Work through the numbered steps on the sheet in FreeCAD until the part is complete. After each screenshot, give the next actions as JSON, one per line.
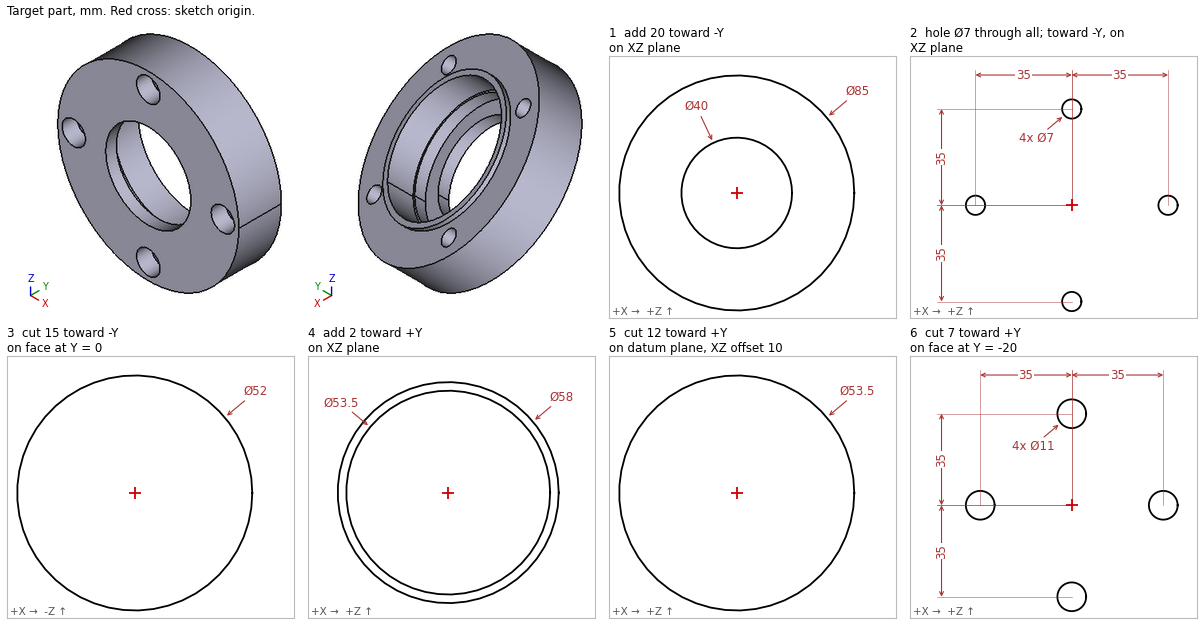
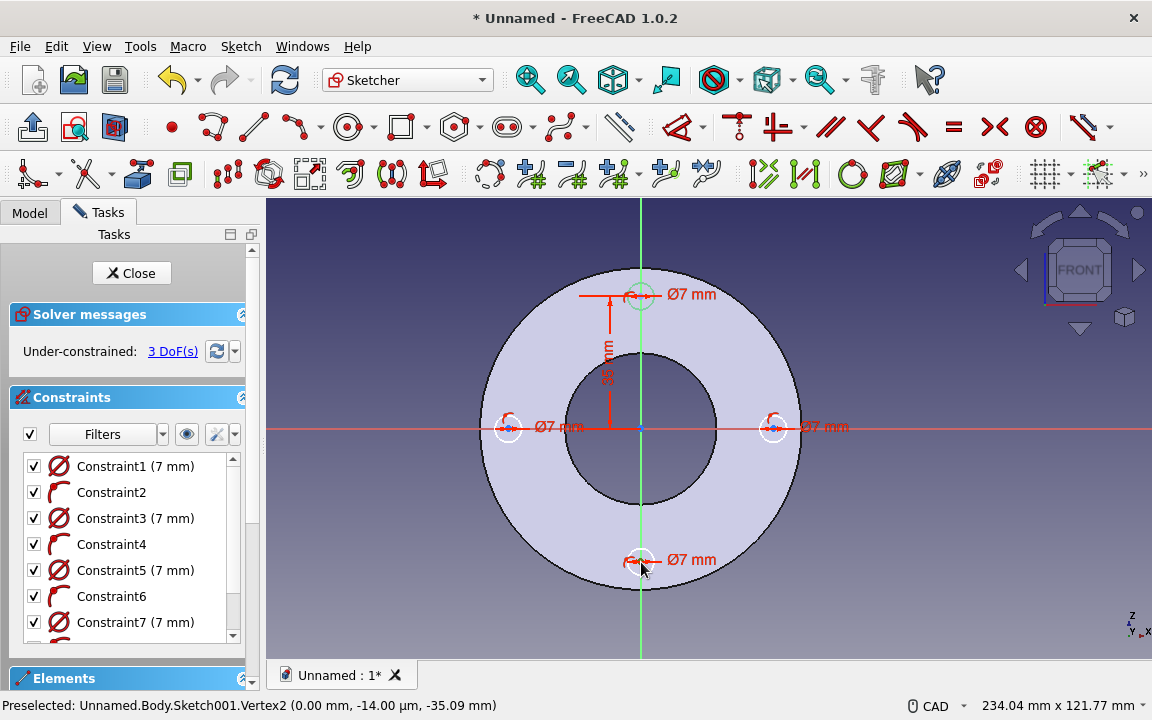
{"action": "key", "text": "i"}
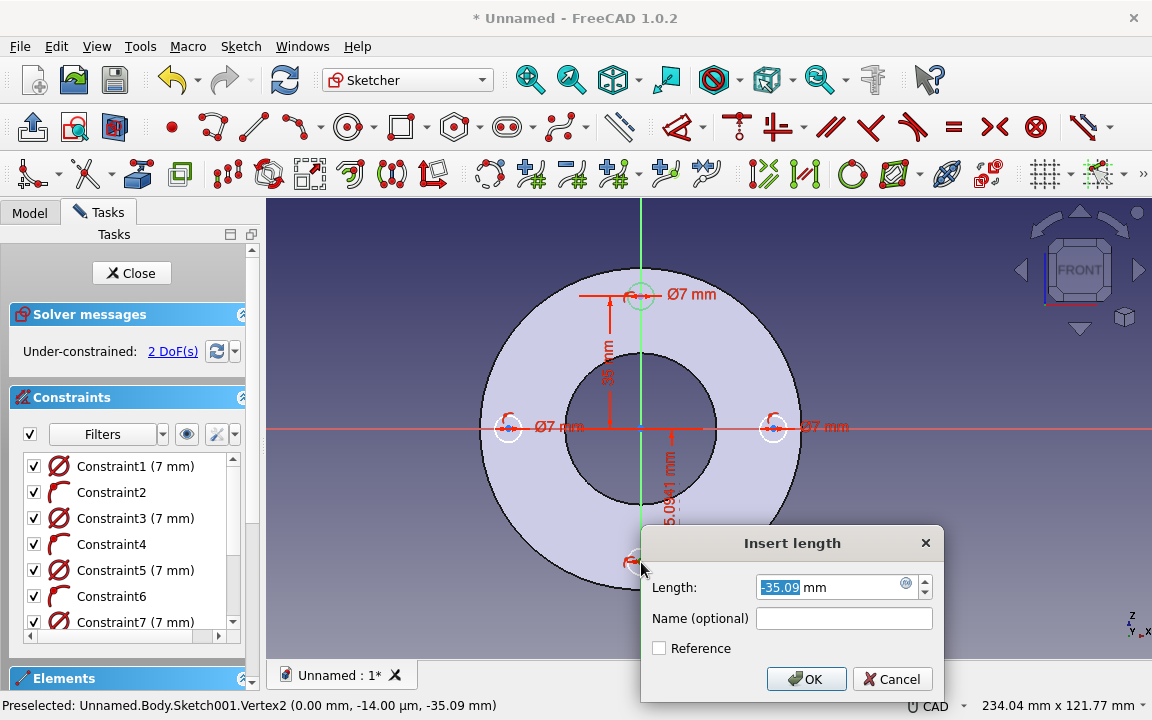
{"action": "type", "text": "-35"}
{"action": "key", "text": "Return"}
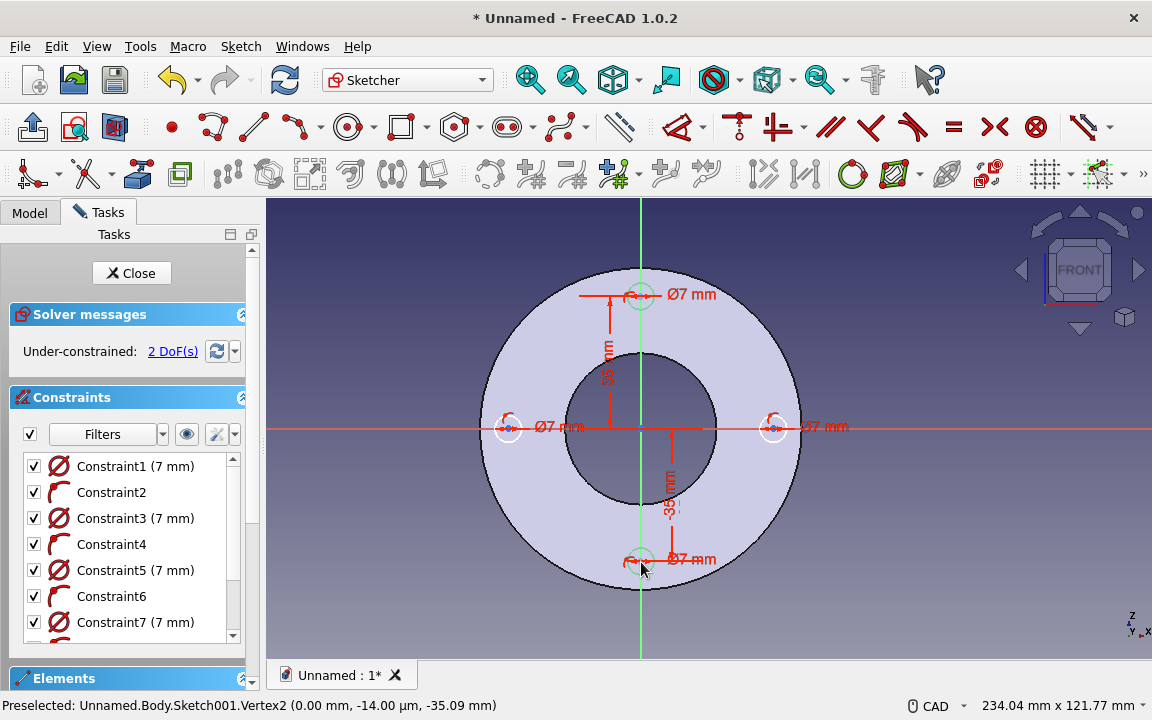
{"action": "left_click", "coordinate": [508, 429]}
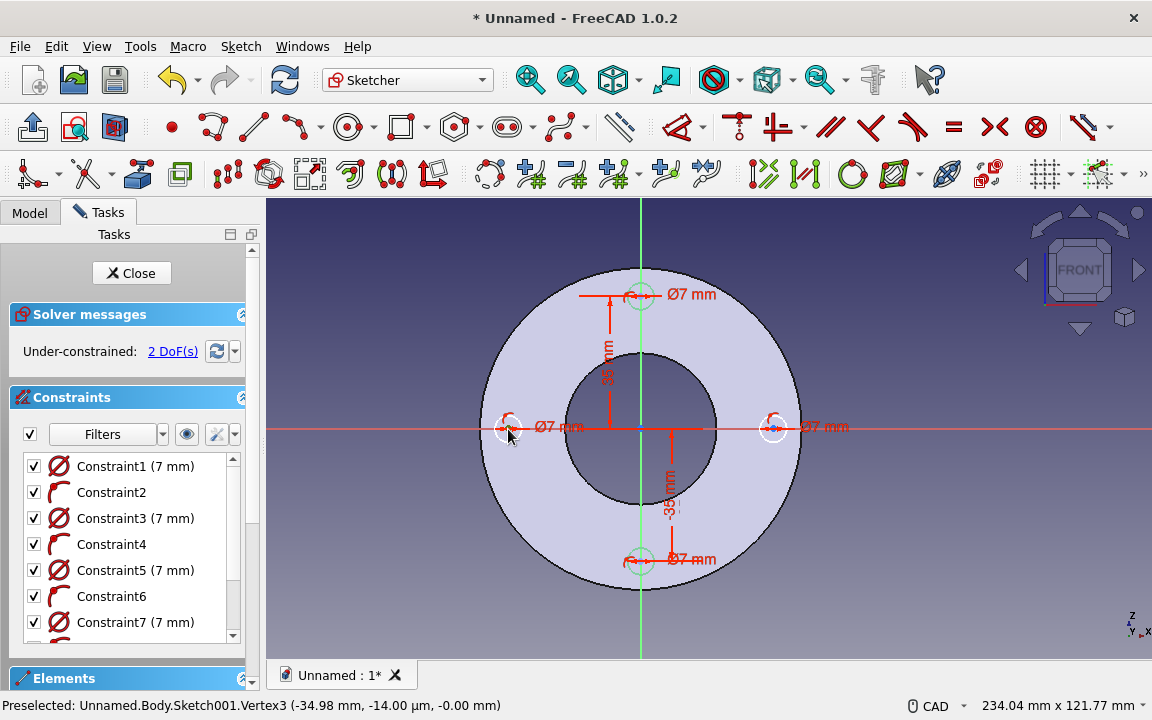
{"action": "key", "text": "l"}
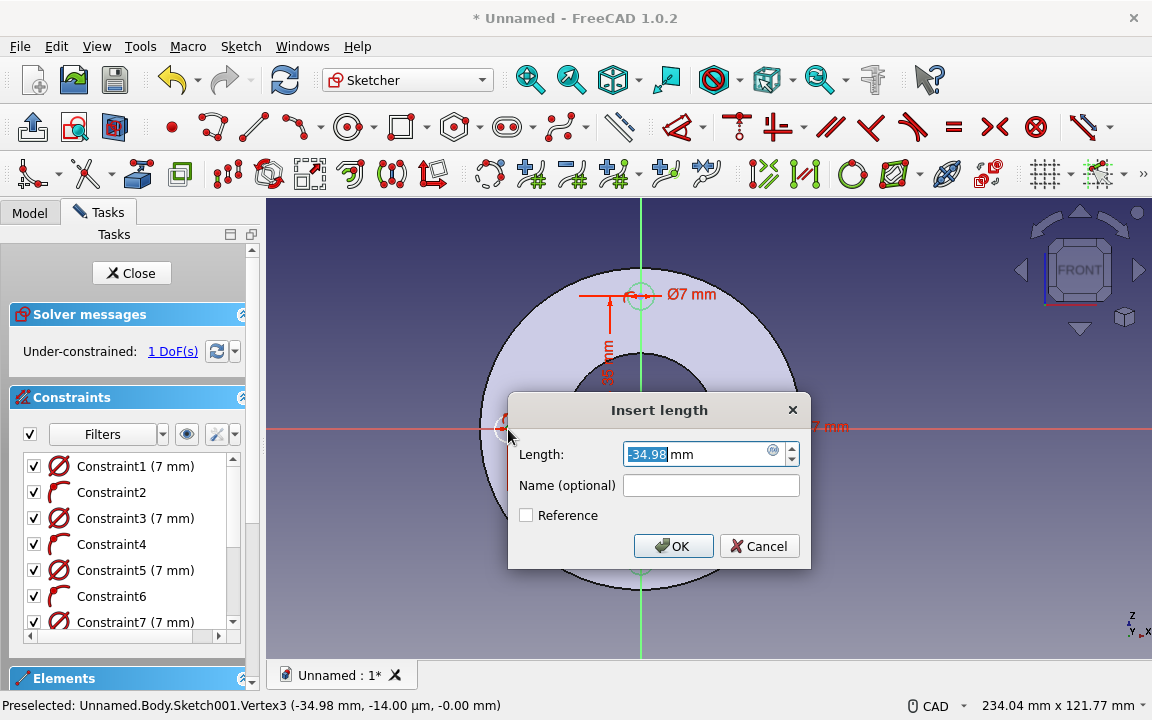
{"action": "type", "text": "-35"}
{"action": "key", "text": "Return"}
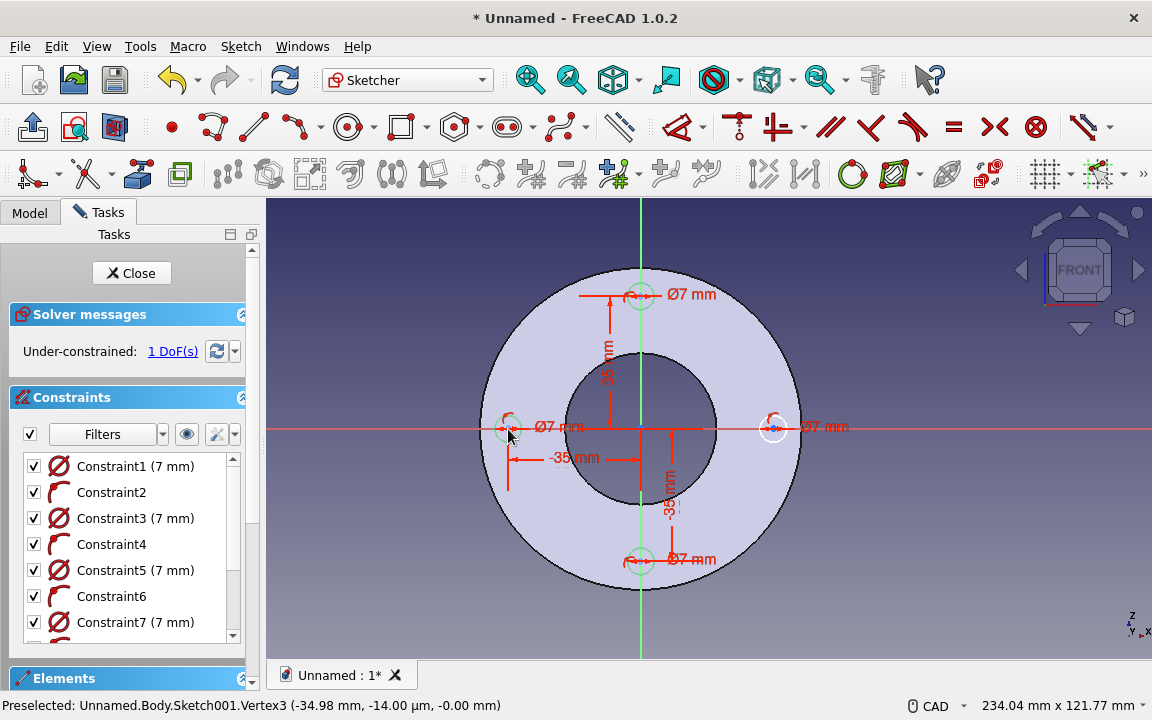
{"action": "left_click", "coordinate": [773, 429]}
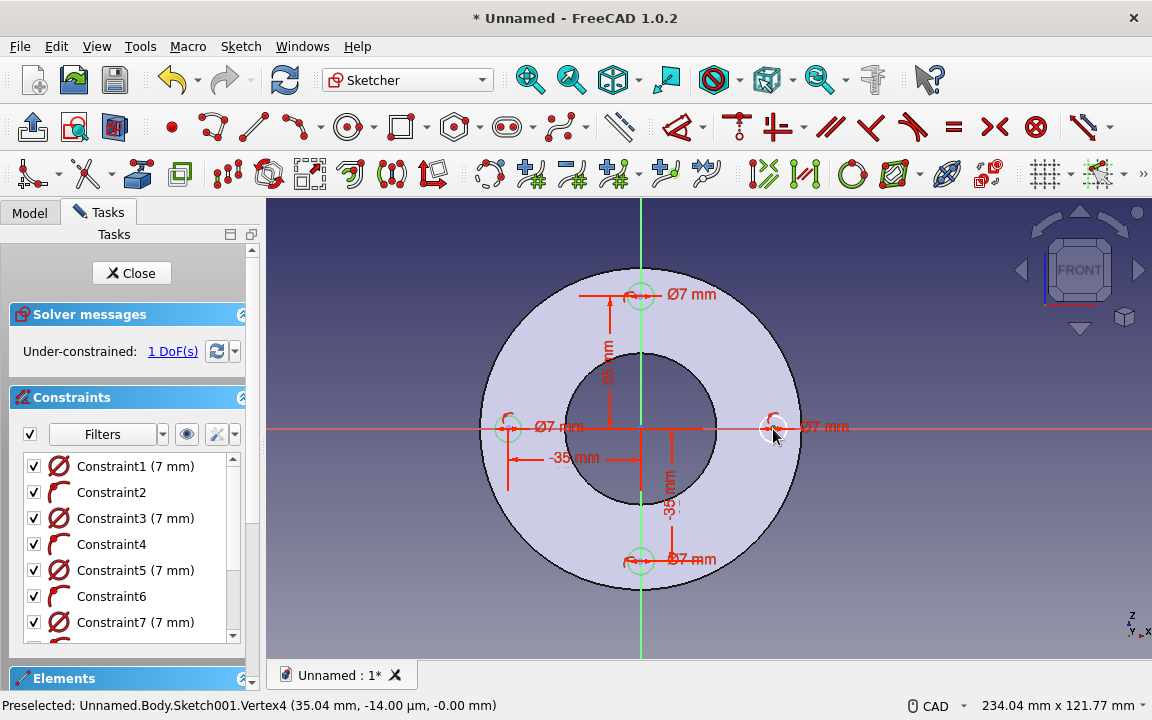
{"action": "key", "text": "l"}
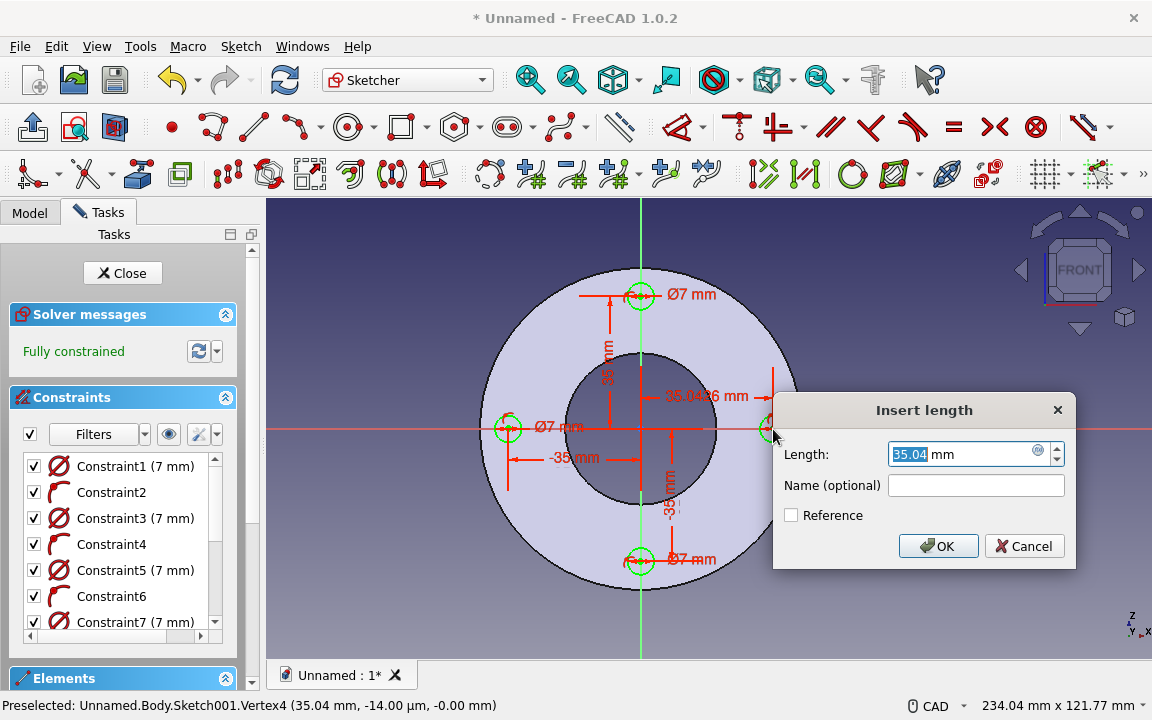
{"action": "type", "text": "35"}
{"action": "key", "text": "Return"}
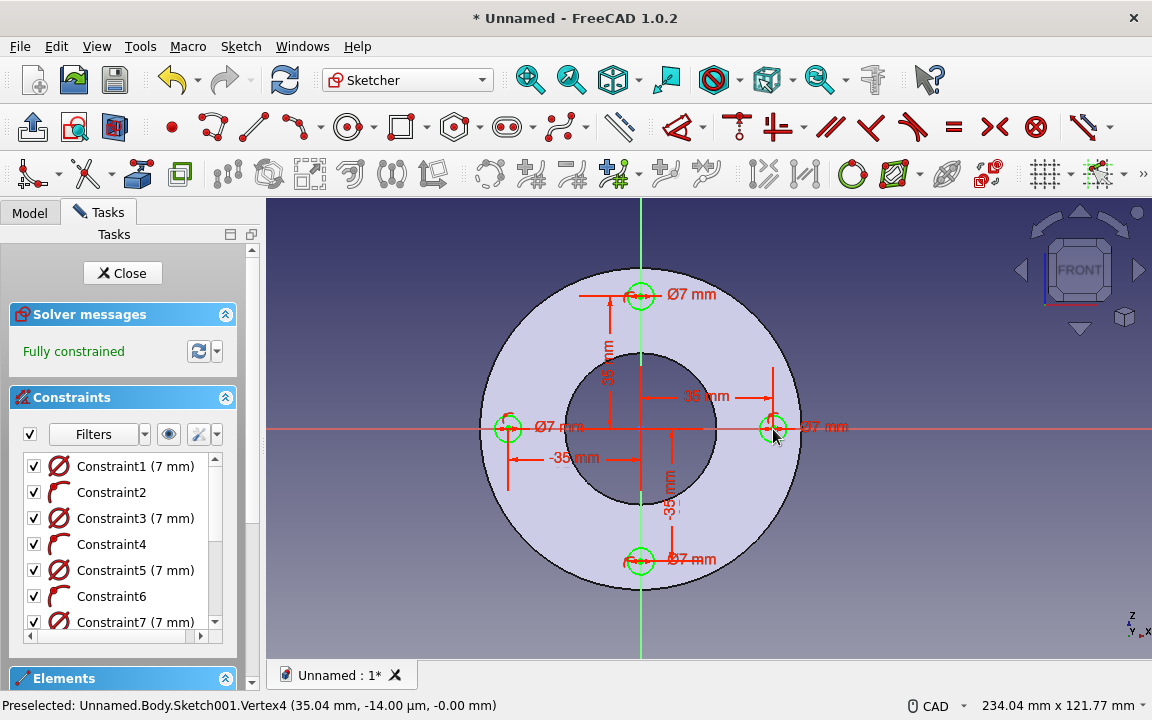
{"action": "left_click", "coordinate": [123, 273]}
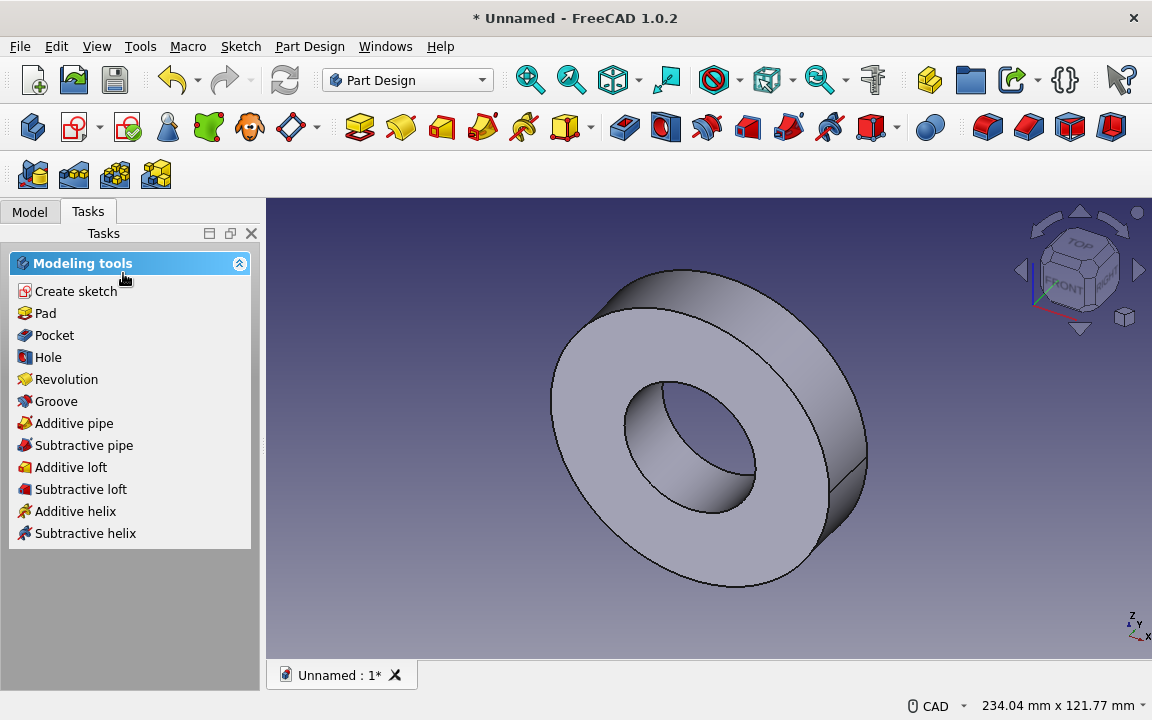
{"action": "left_click", "coordinate": [666, 128]}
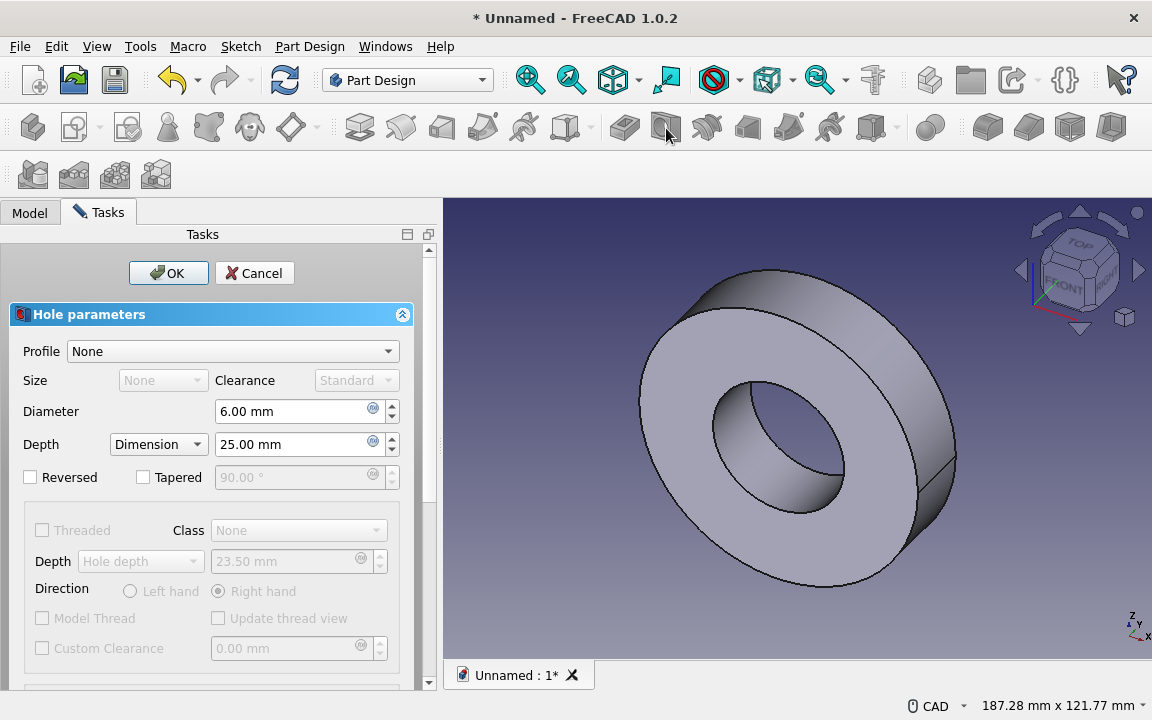
{"action": "triple_click", "coordinate": [300, 412]}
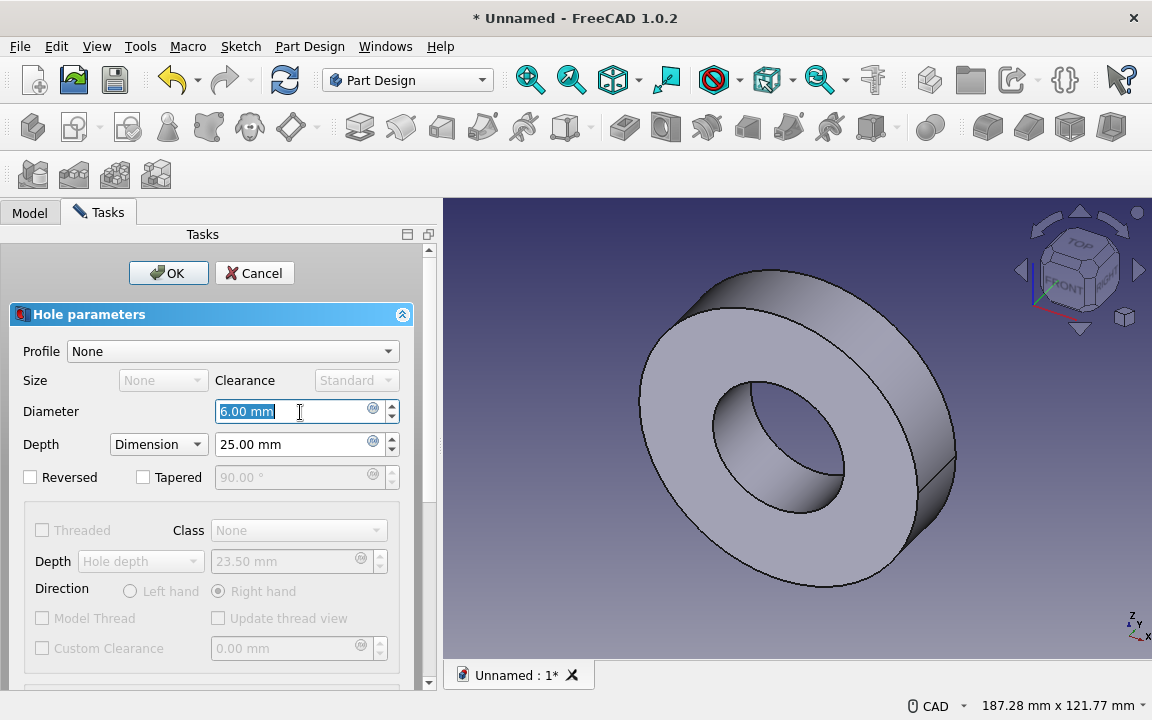
{"action": "type", "text": "7"}
{"action": "key", "text": "Tab"}